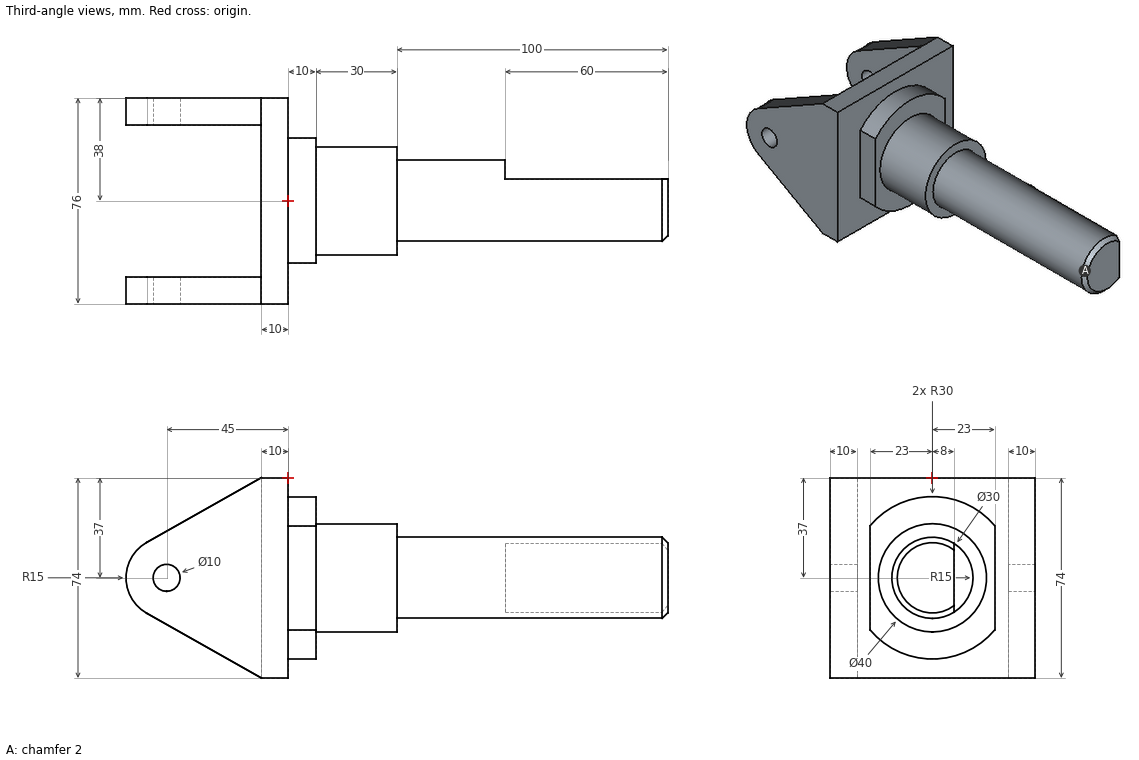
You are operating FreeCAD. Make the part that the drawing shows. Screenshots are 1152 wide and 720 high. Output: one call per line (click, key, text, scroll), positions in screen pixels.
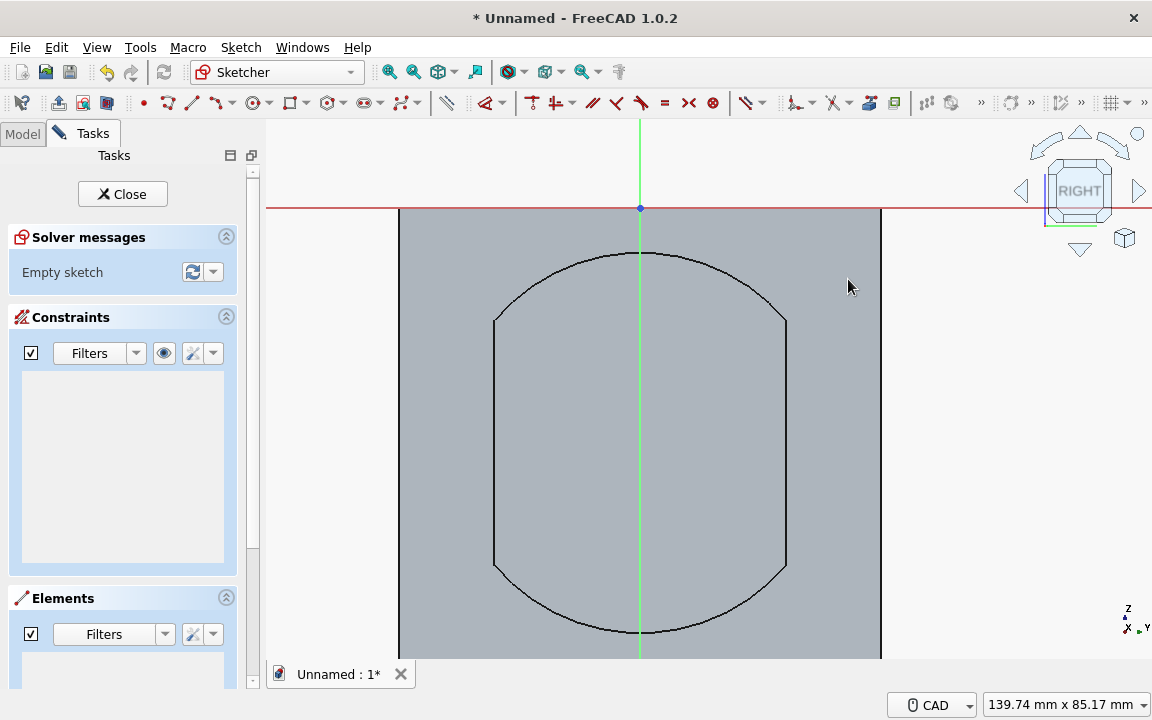
click(254, 104)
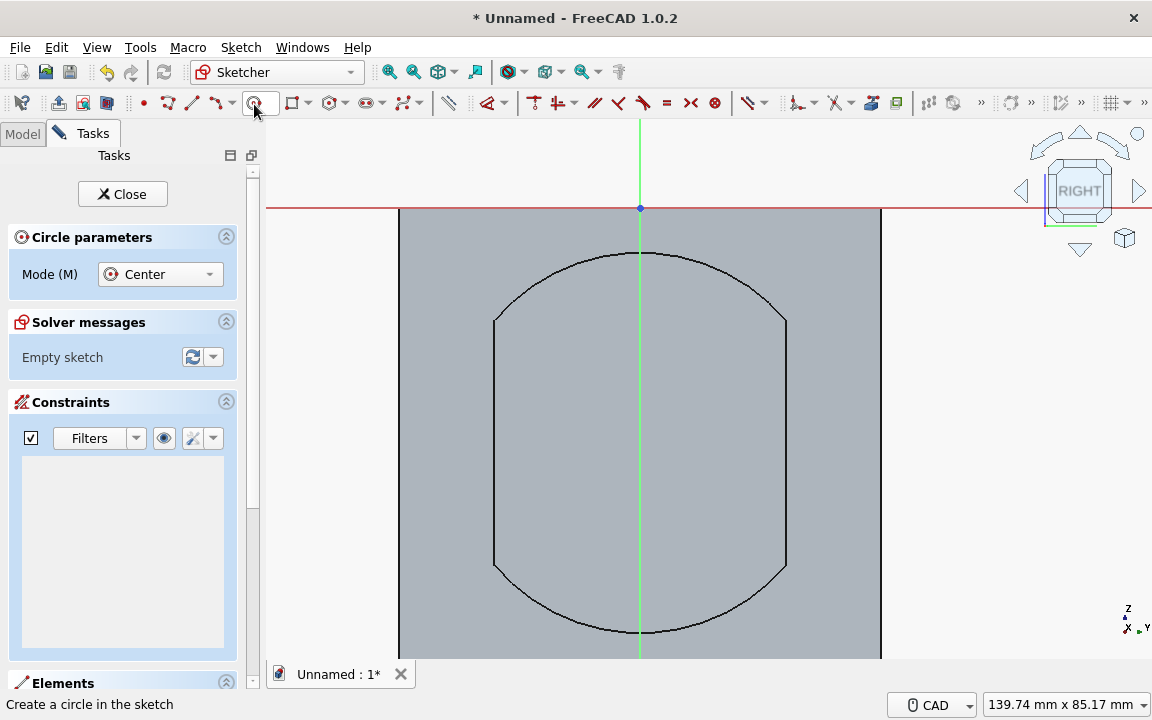
click(640, 443)
click(730, 353)
key(Escape)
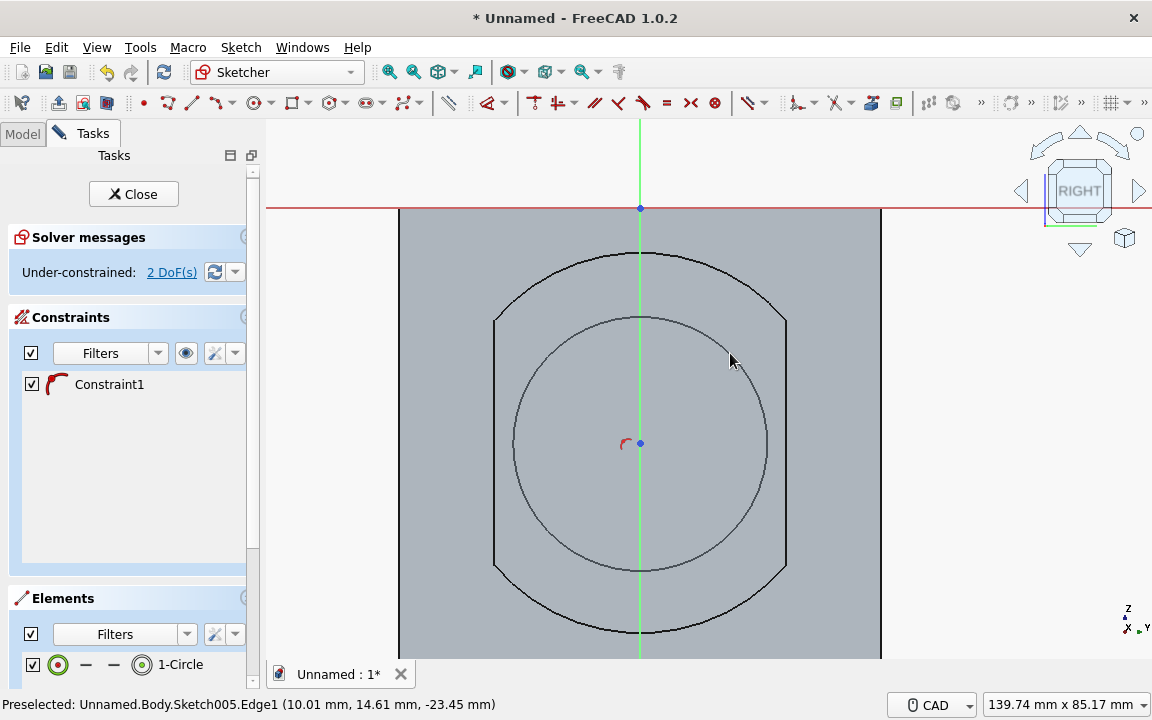
click(488, 104)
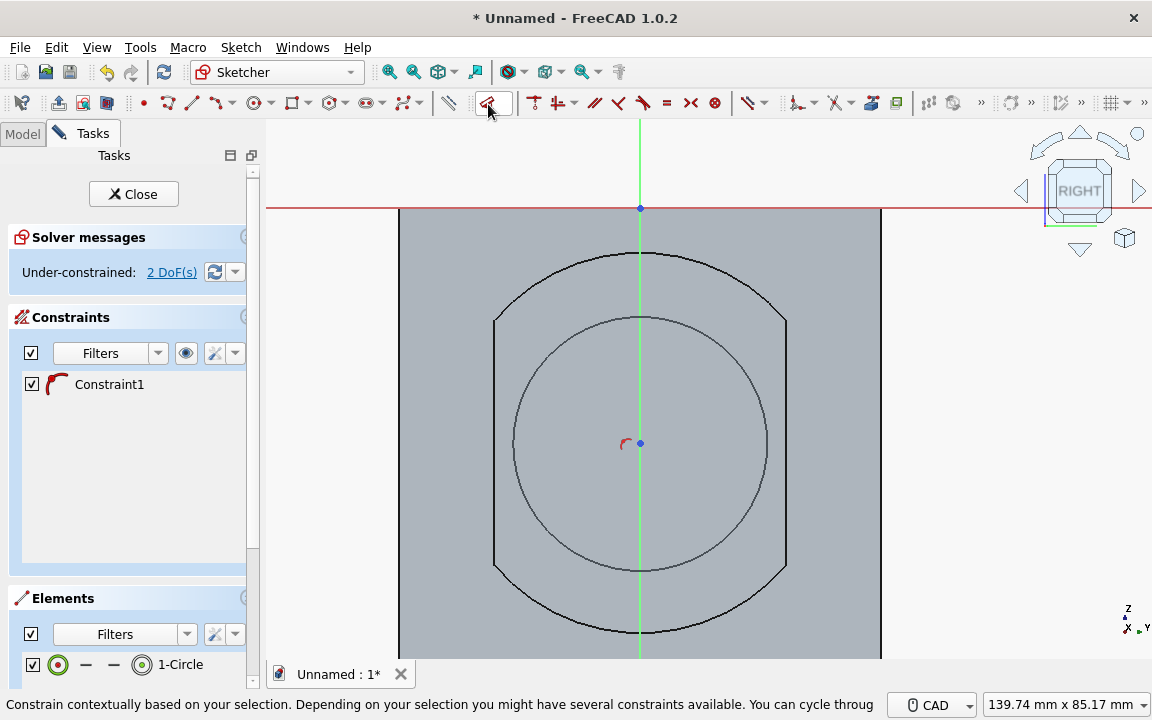
click(730, 354)
click(753, 331)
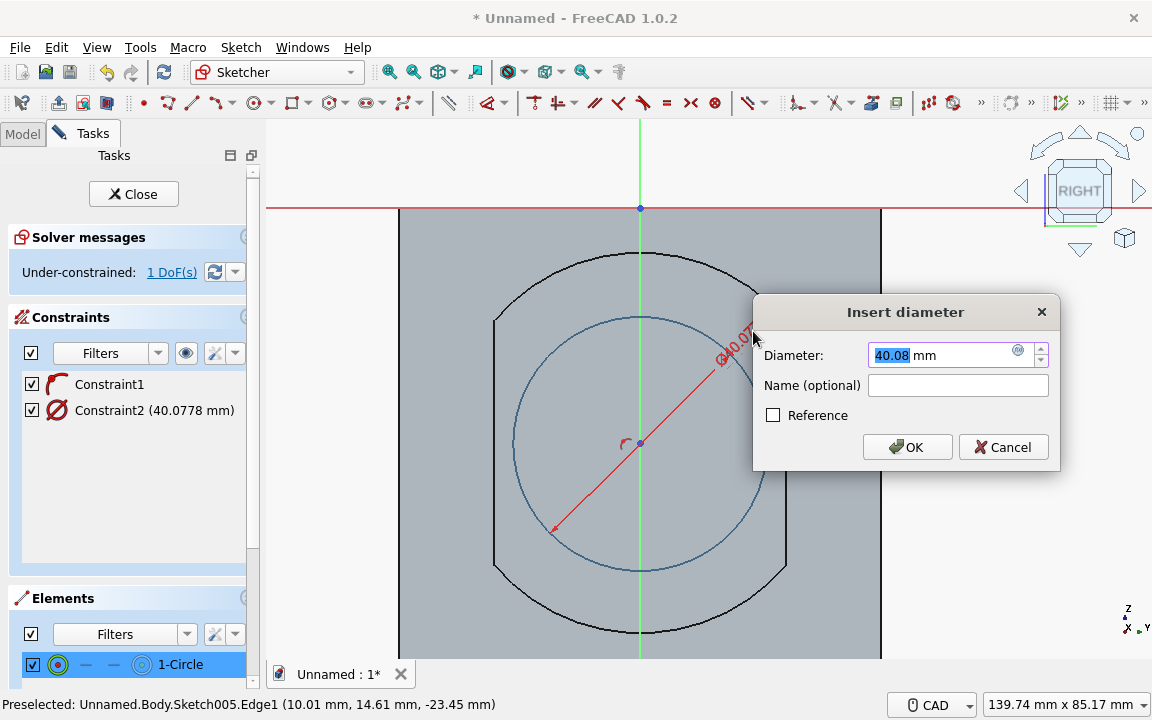
text(40)
key(Return)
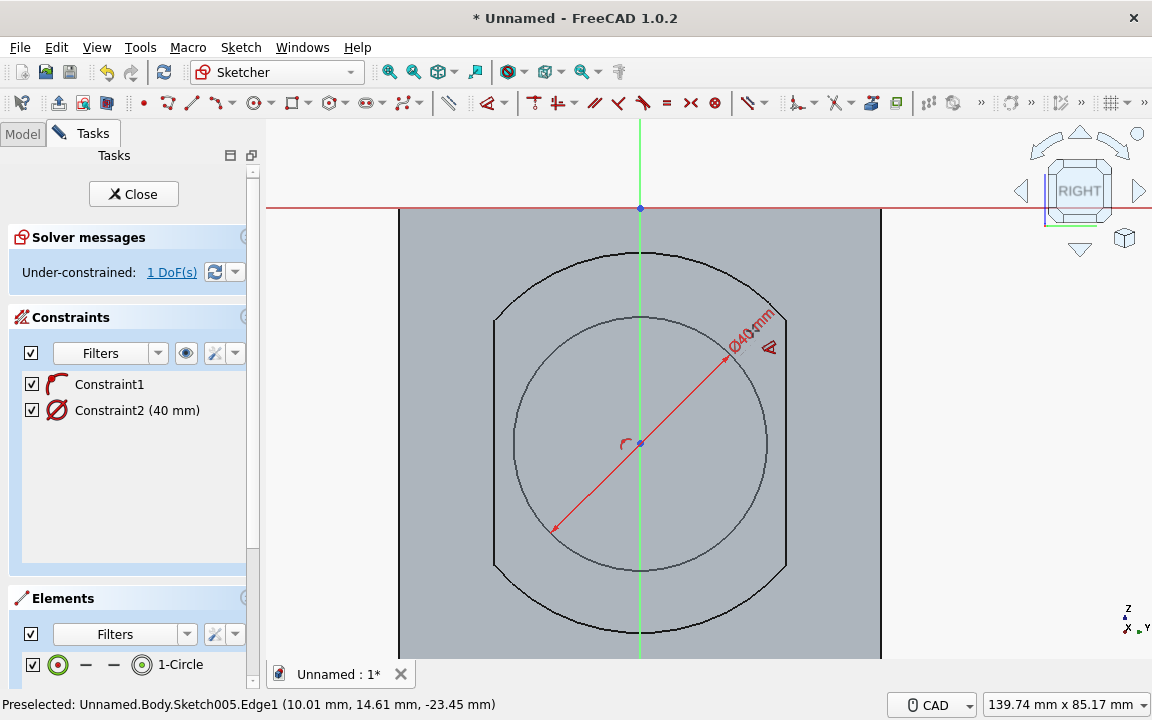
click(640, 444)
click(674, 272)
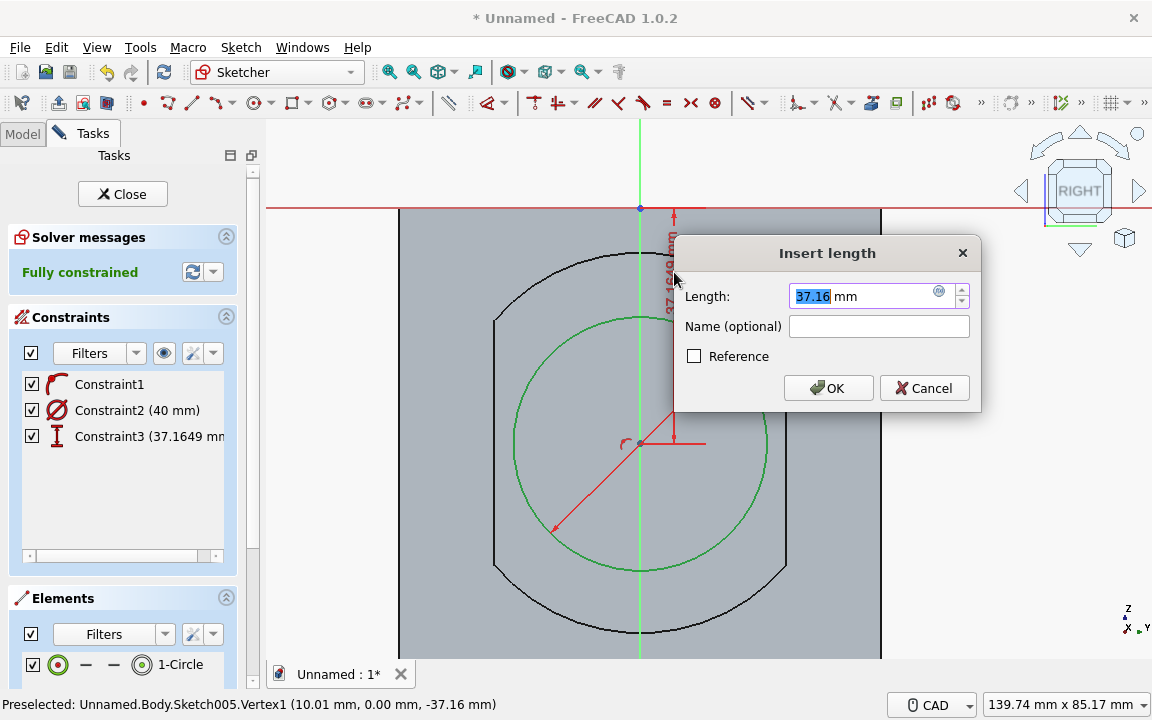
text(37)
key(Return)
key(Escape)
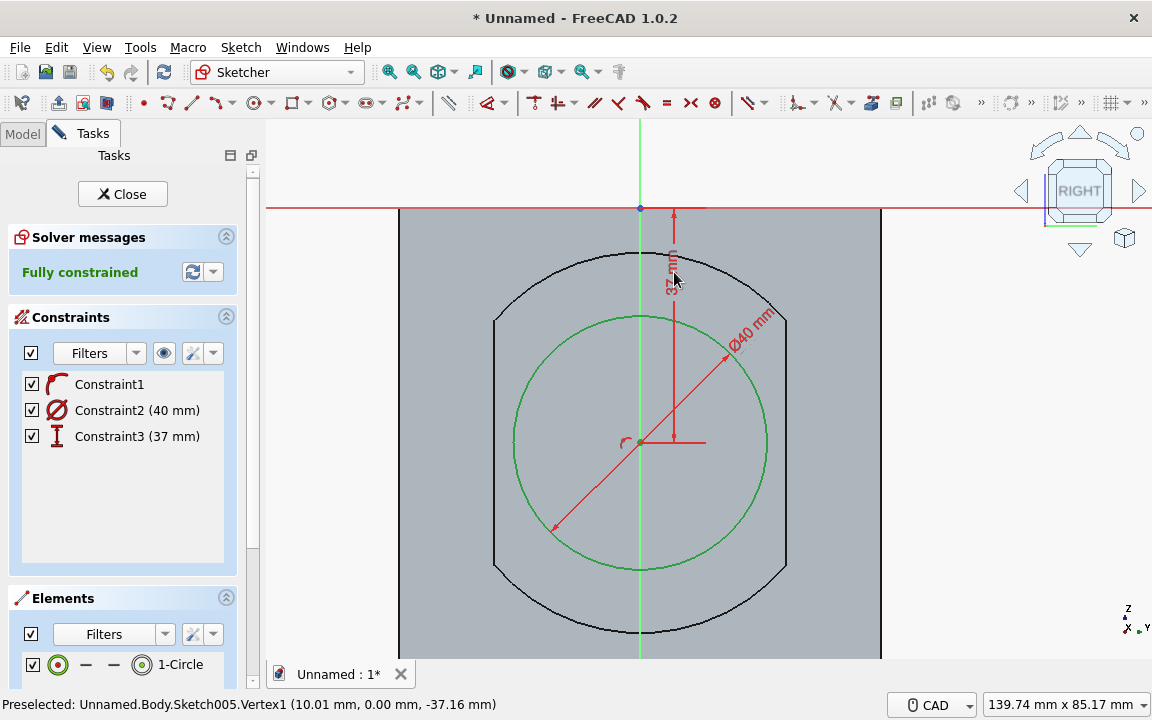
click(123, 194)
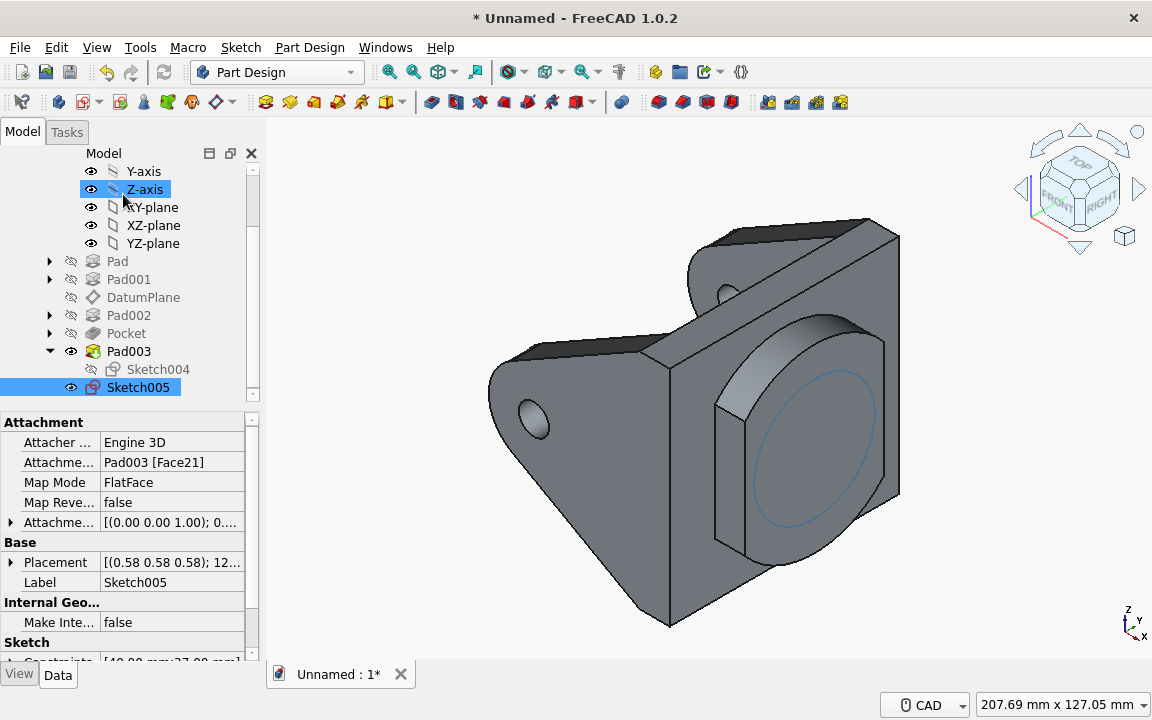
click(266, 102)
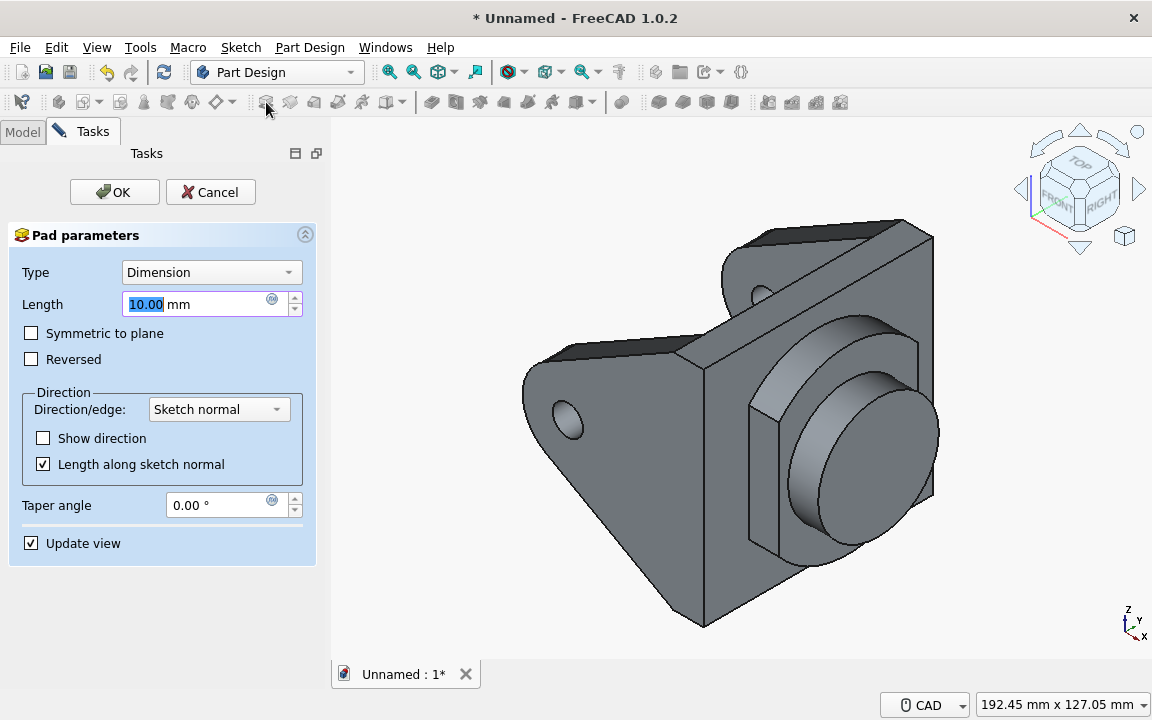
text(30)
key(Tab)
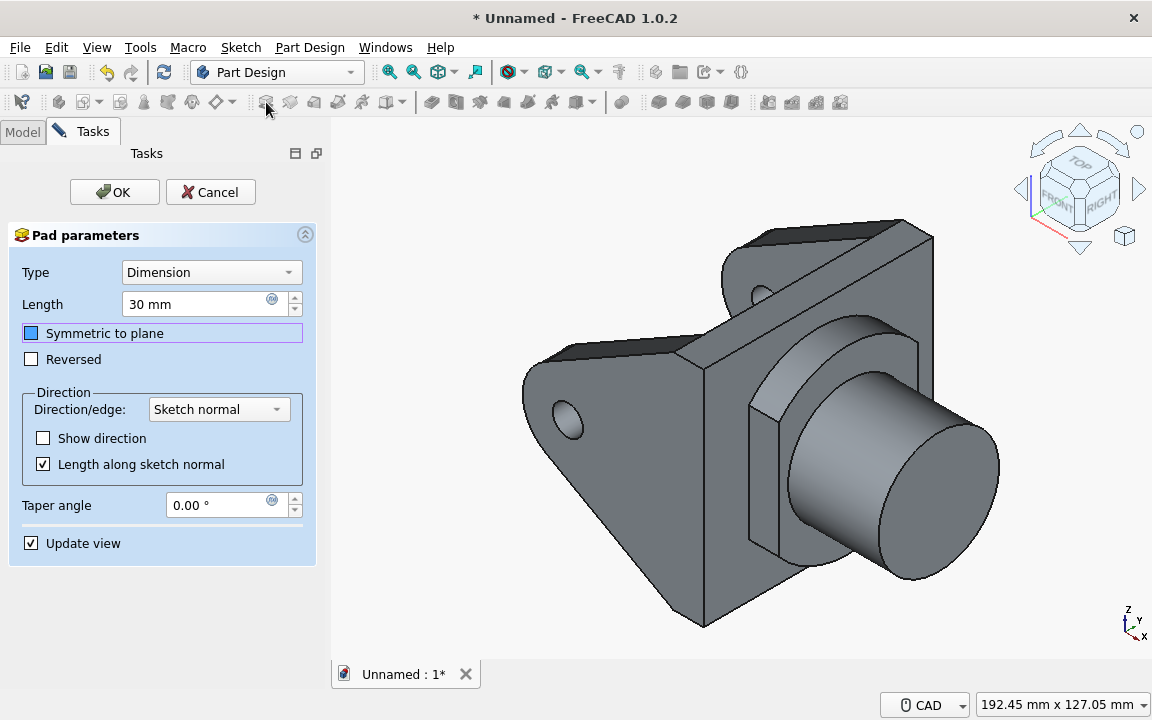
click(115, 192)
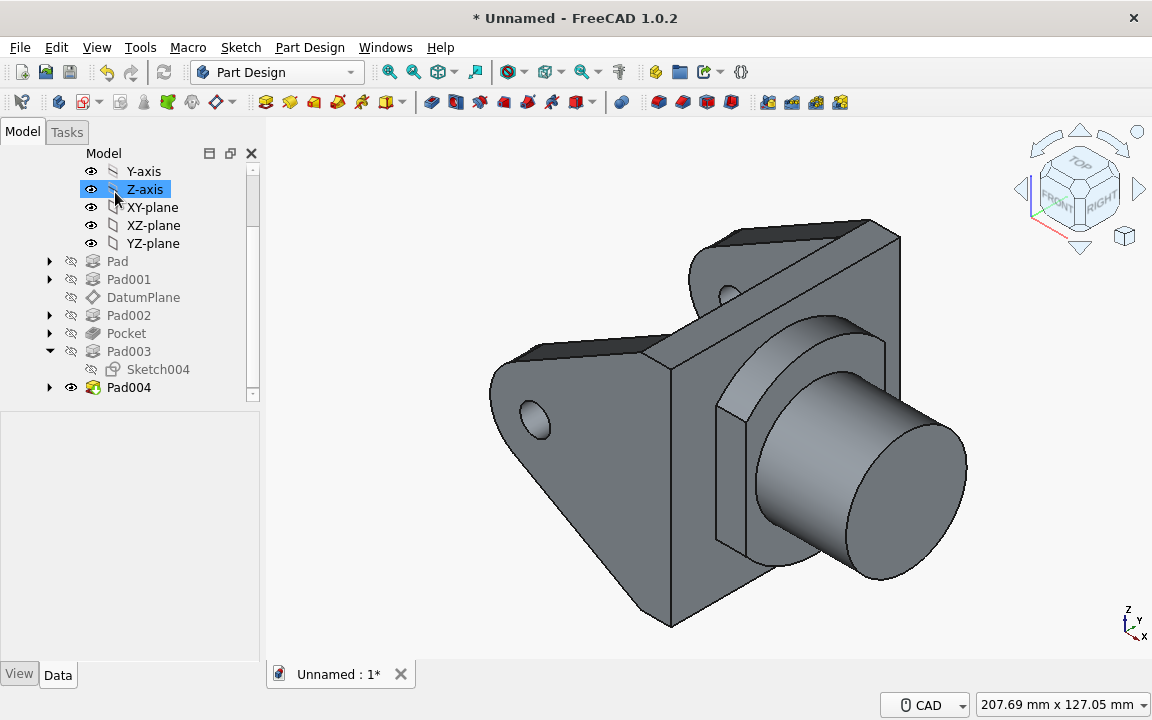
click(390, 72)